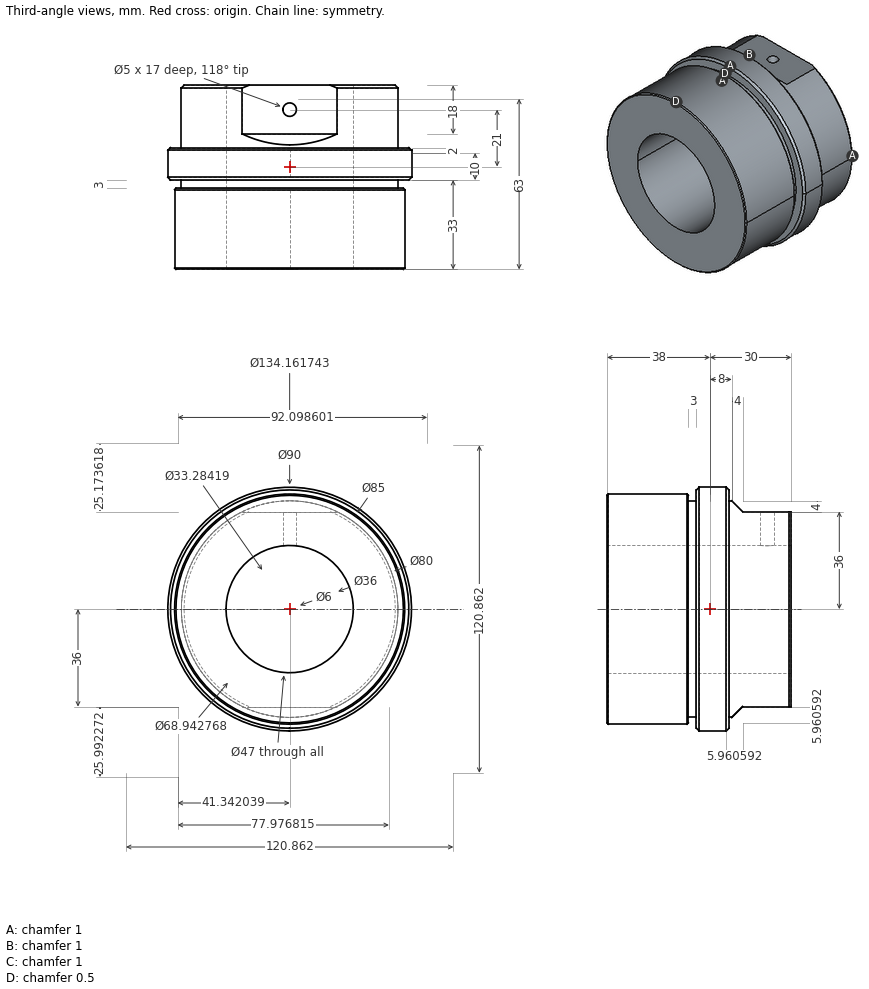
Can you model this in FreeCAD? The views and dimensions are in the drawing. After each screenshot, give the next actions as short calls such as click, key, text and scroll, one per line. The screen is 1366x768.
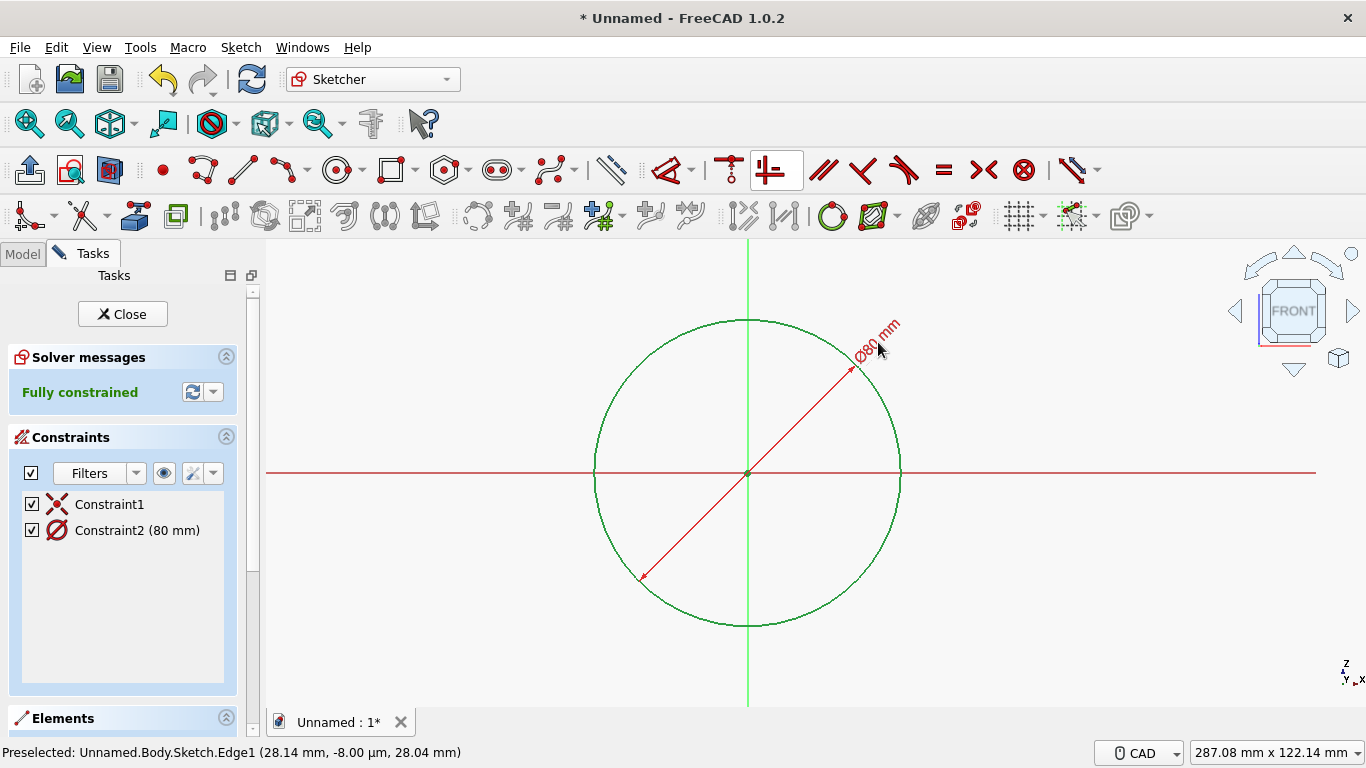
click(123, 314)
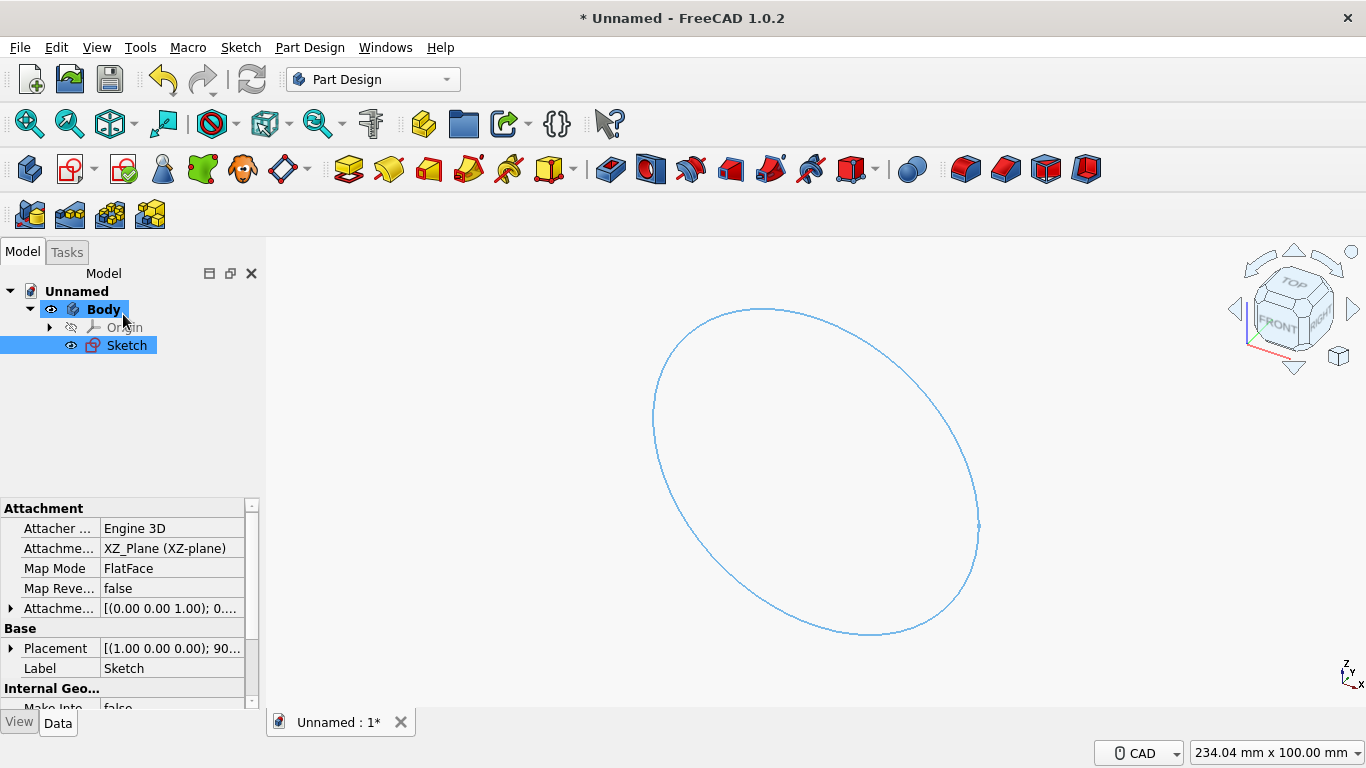
click(350, 170)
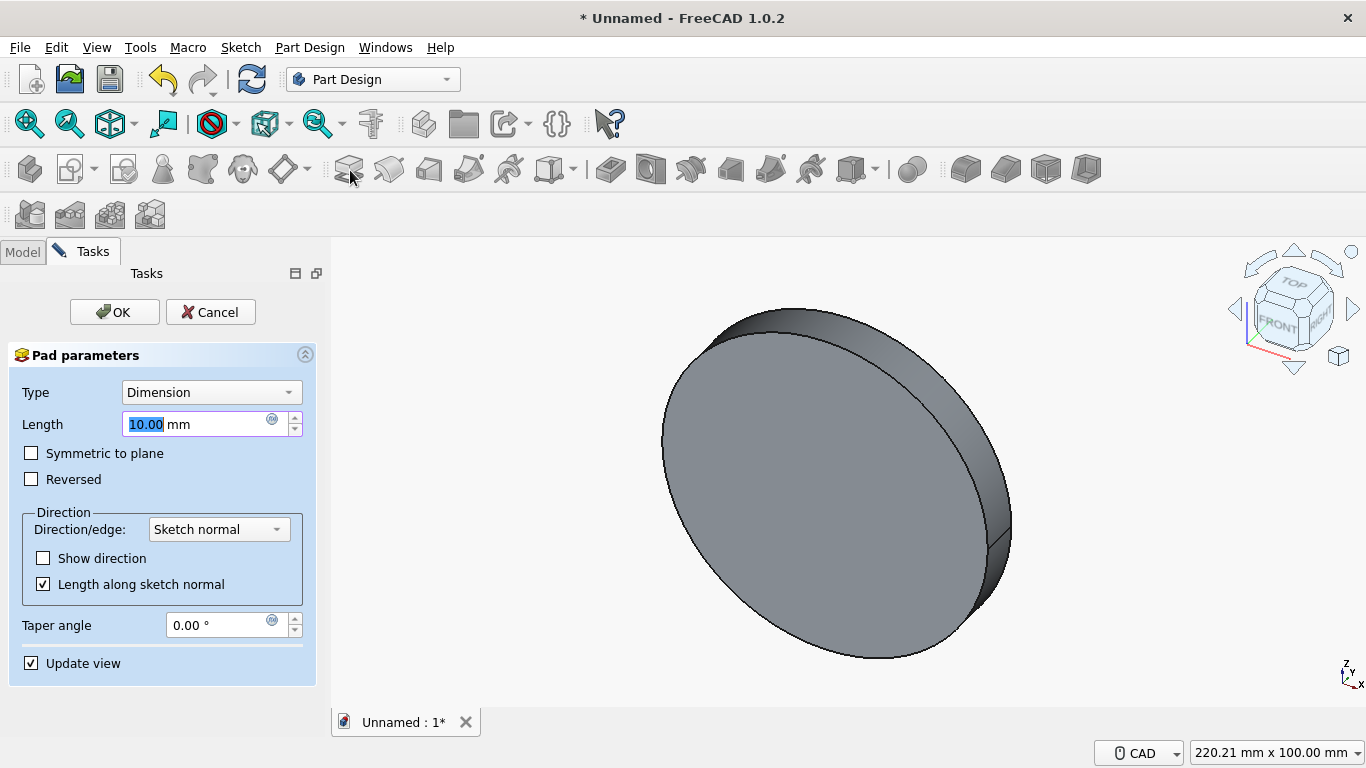
text(30)
key(Tab)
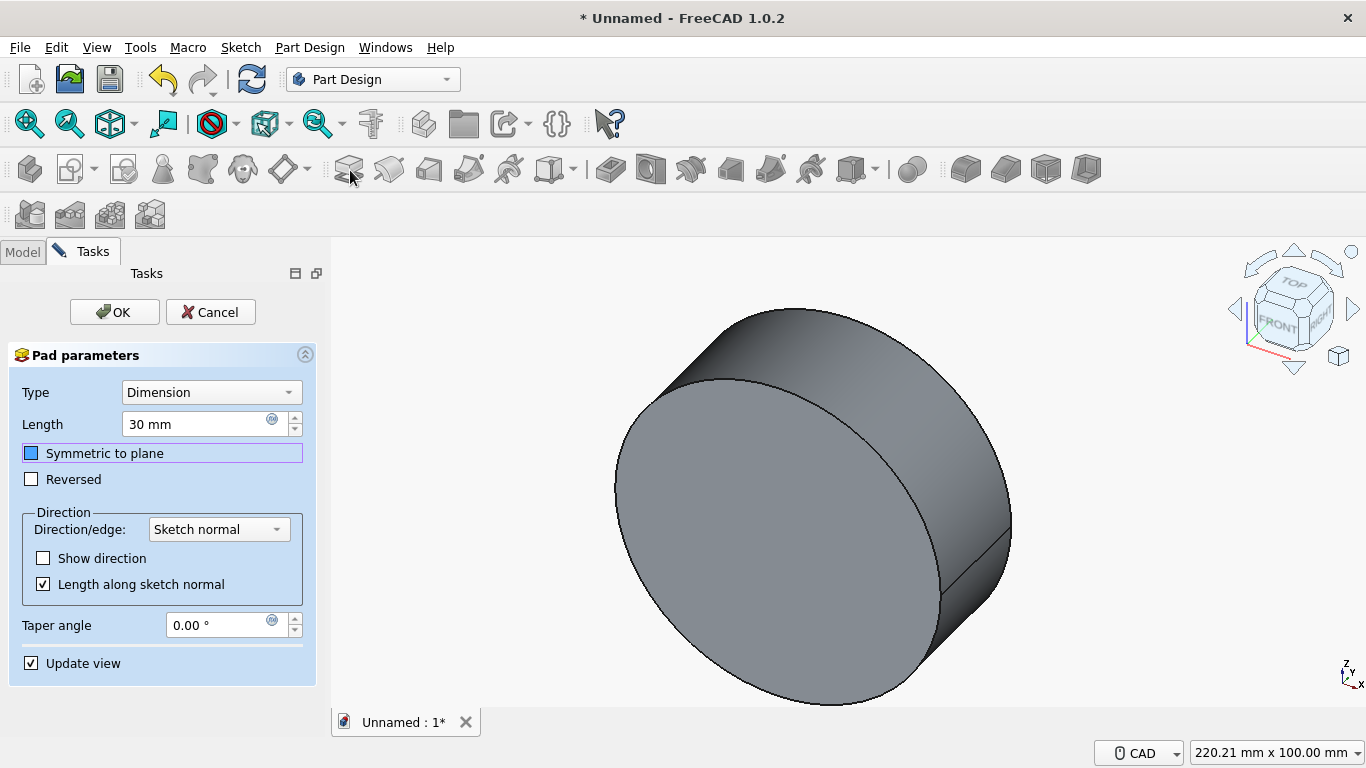
click(30, 479)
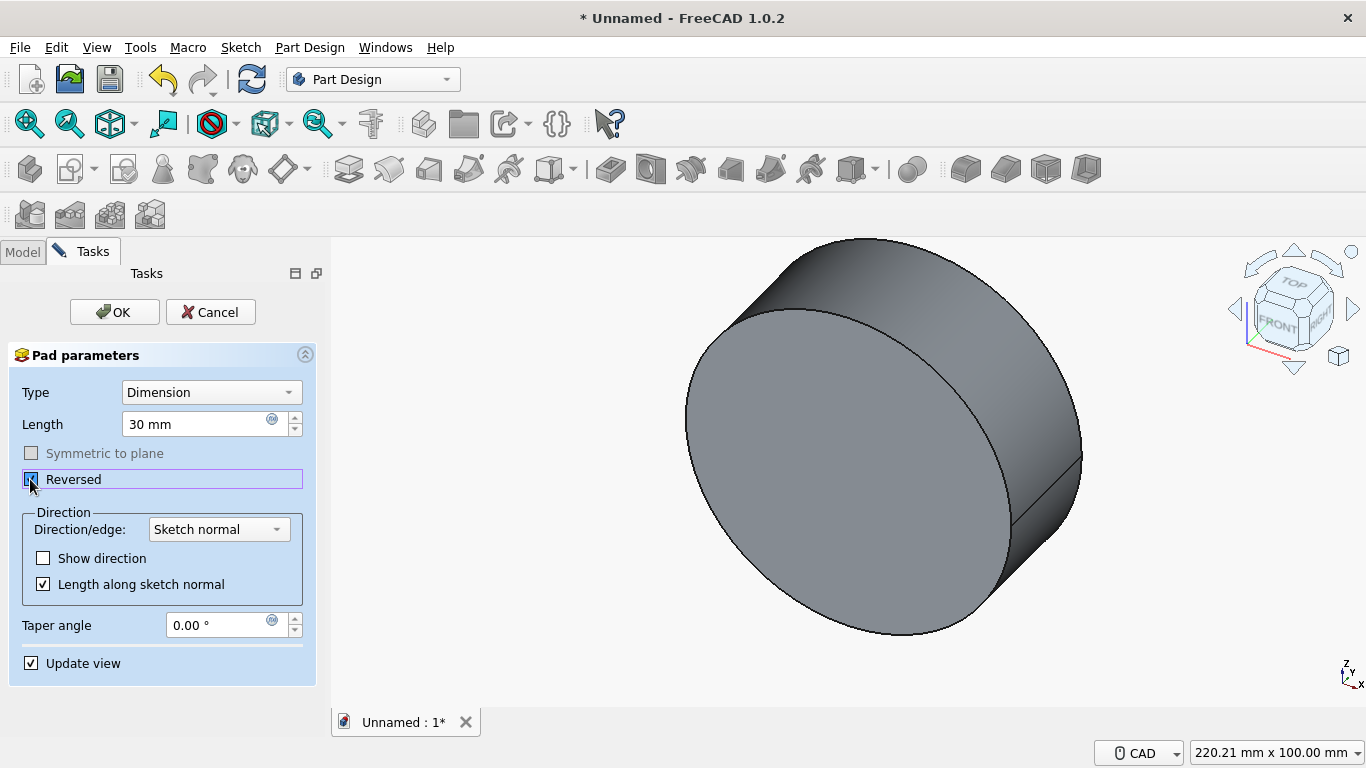
click(115, 312)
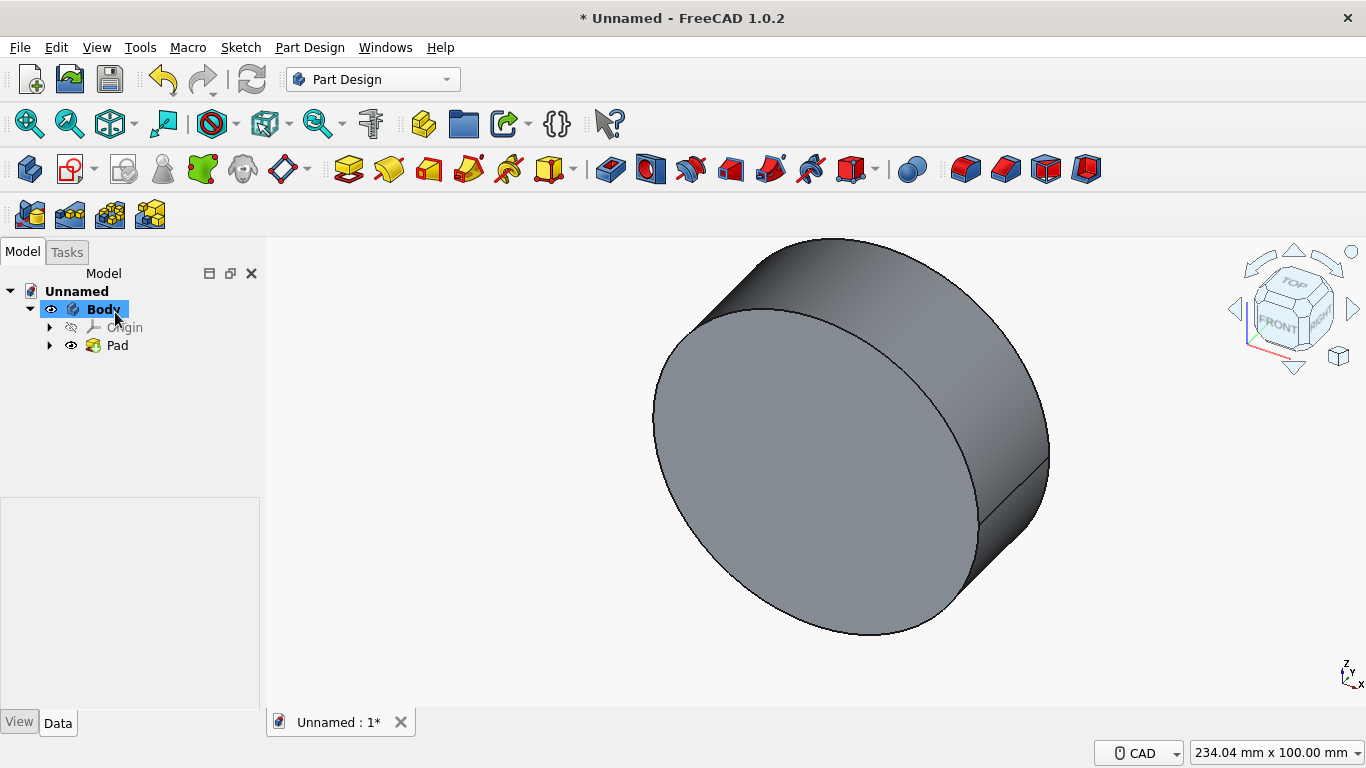
click(30, 124)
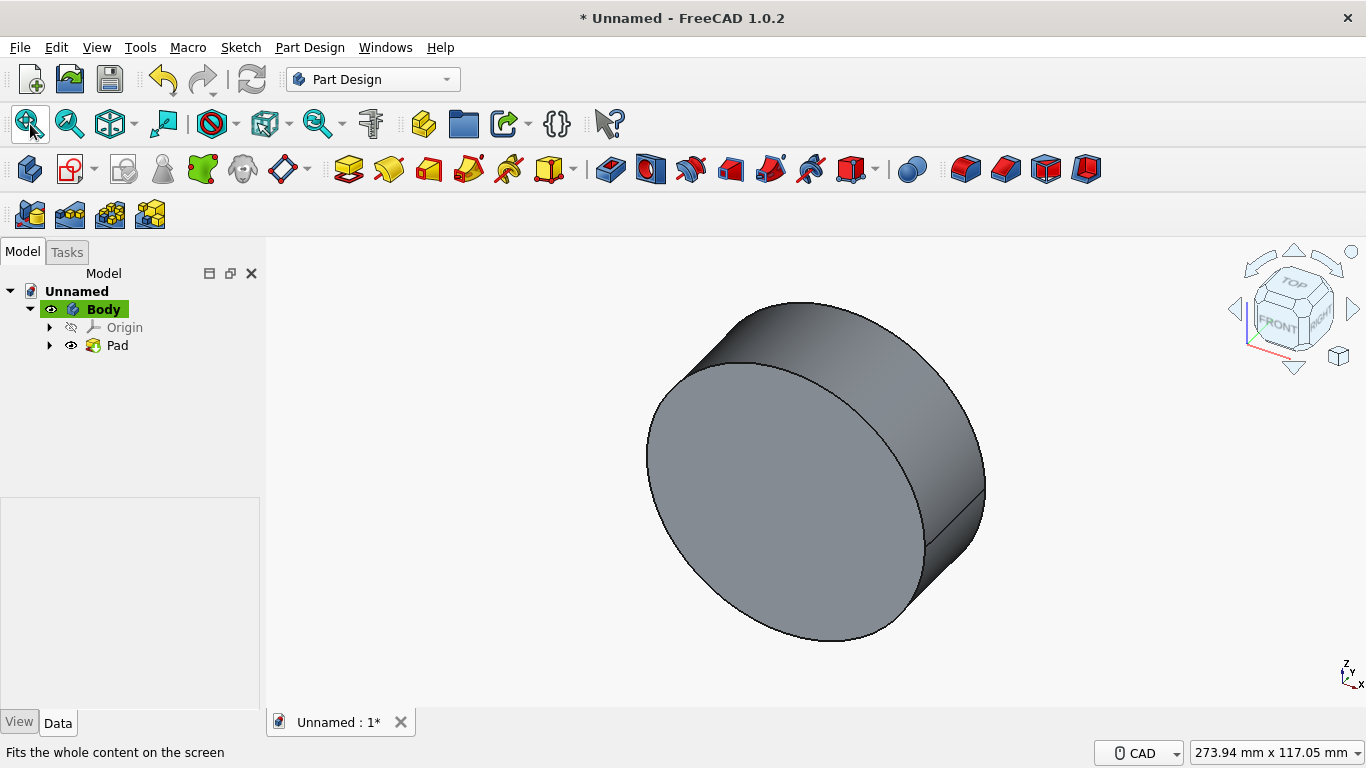
key(4)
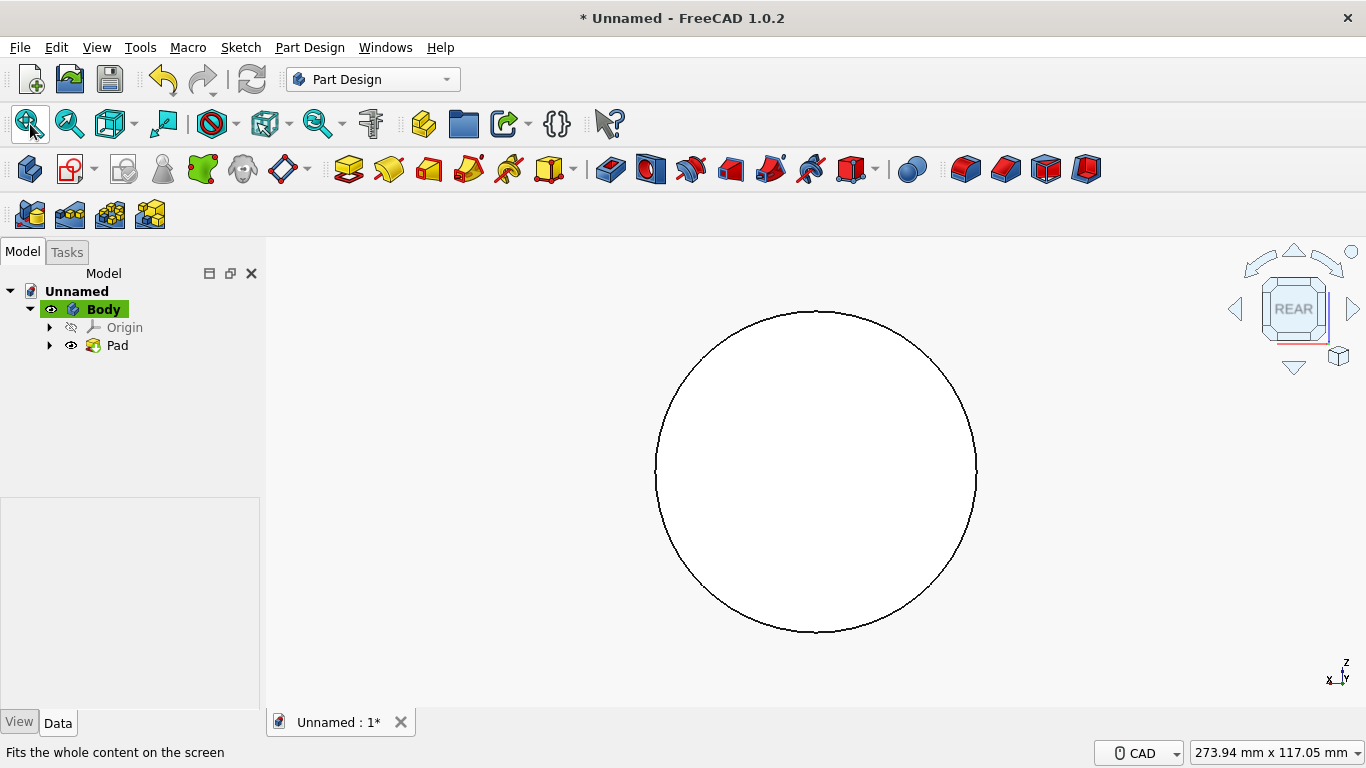
click(816, 471)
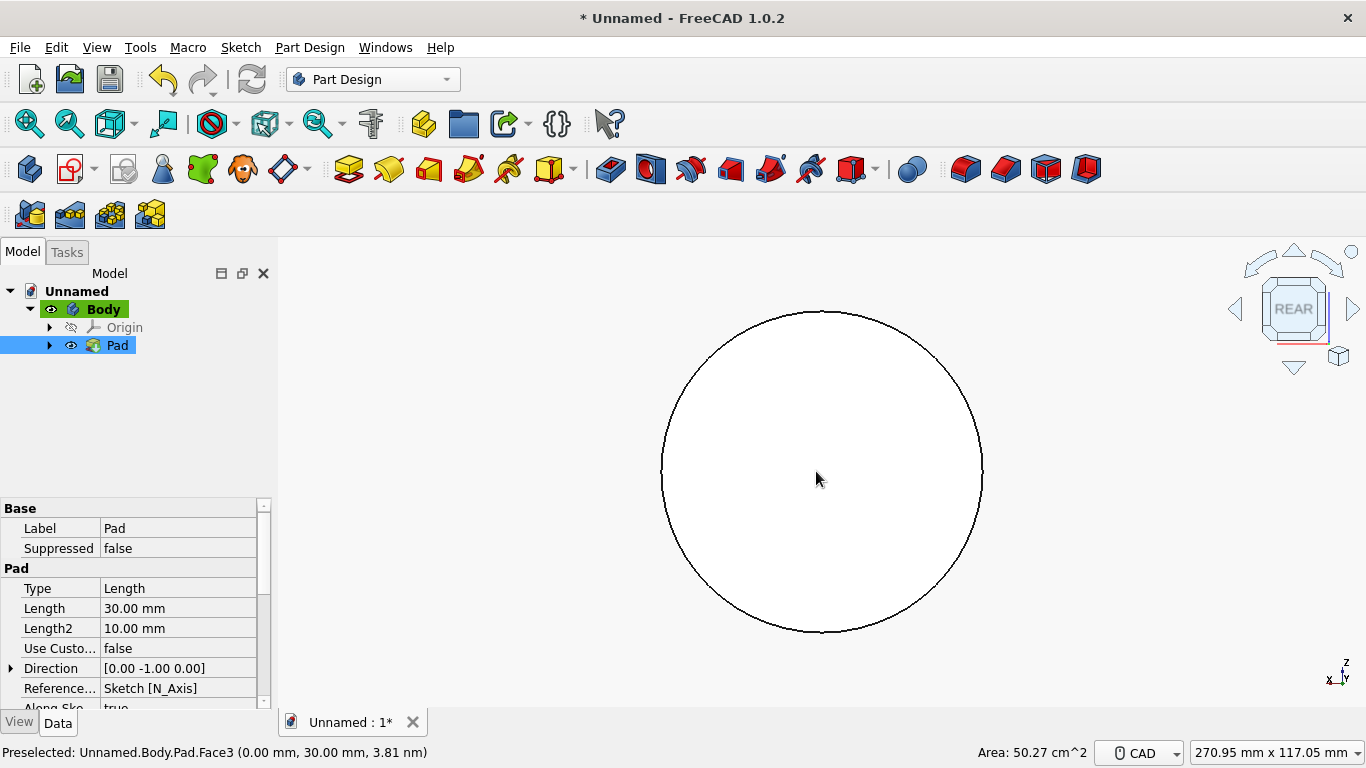
click(70, 170)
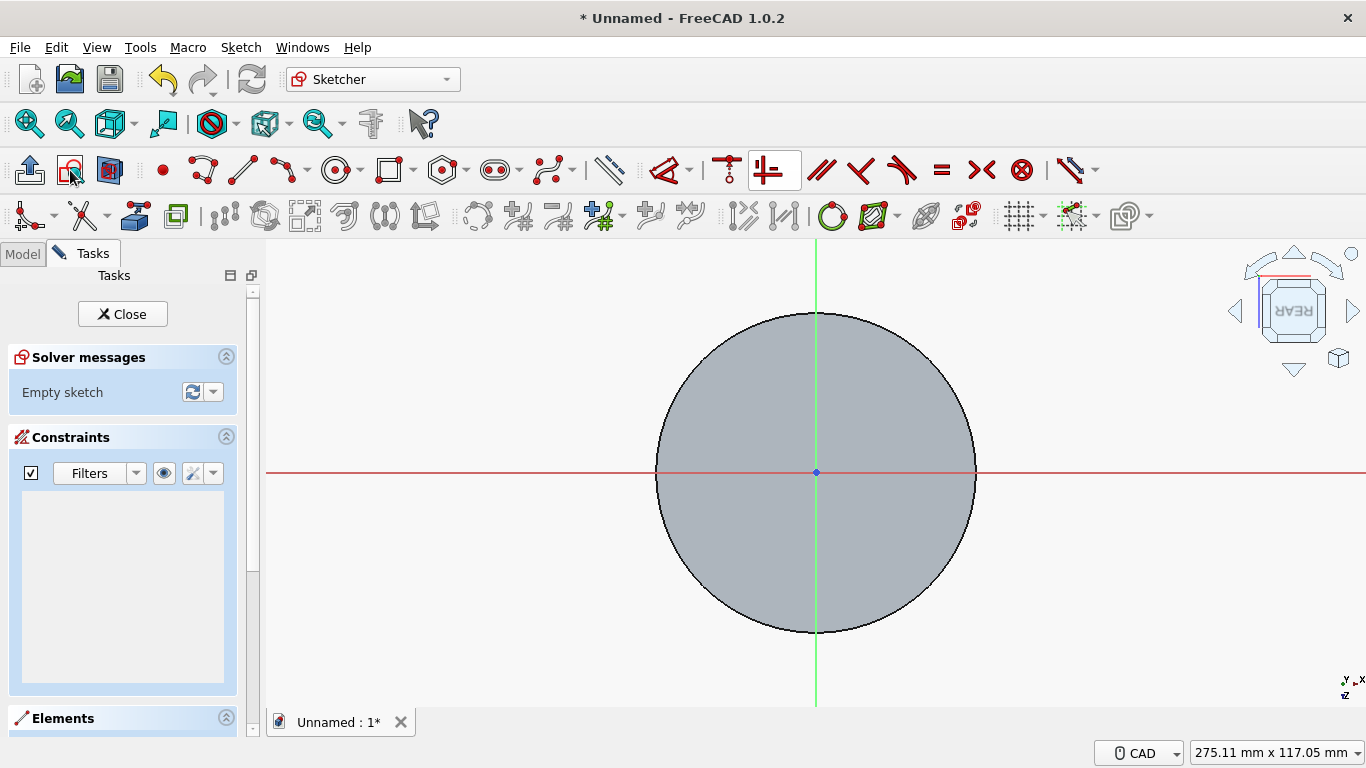
scroll(872, 473, up, 4)